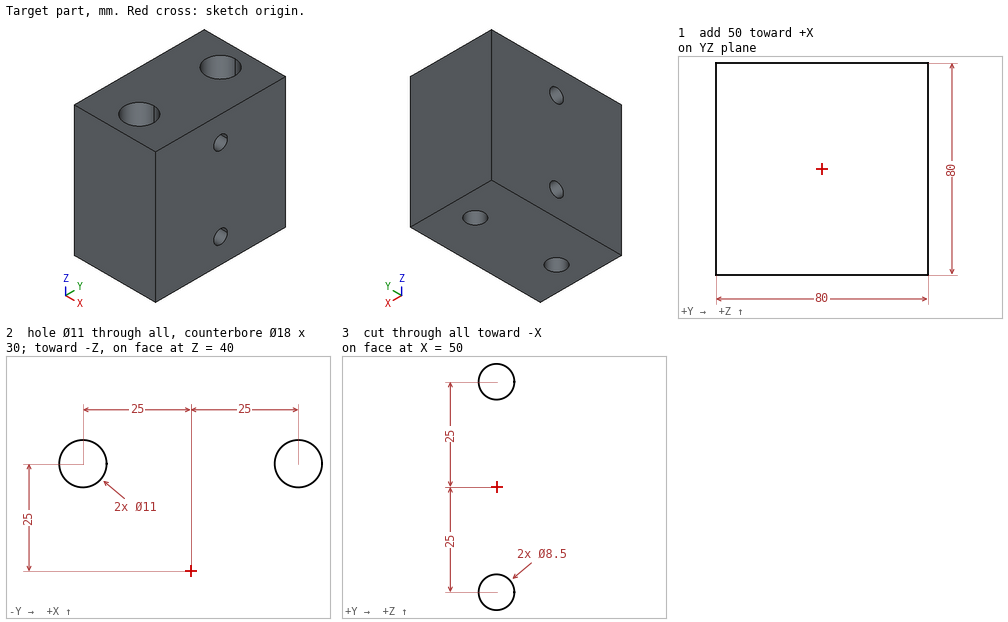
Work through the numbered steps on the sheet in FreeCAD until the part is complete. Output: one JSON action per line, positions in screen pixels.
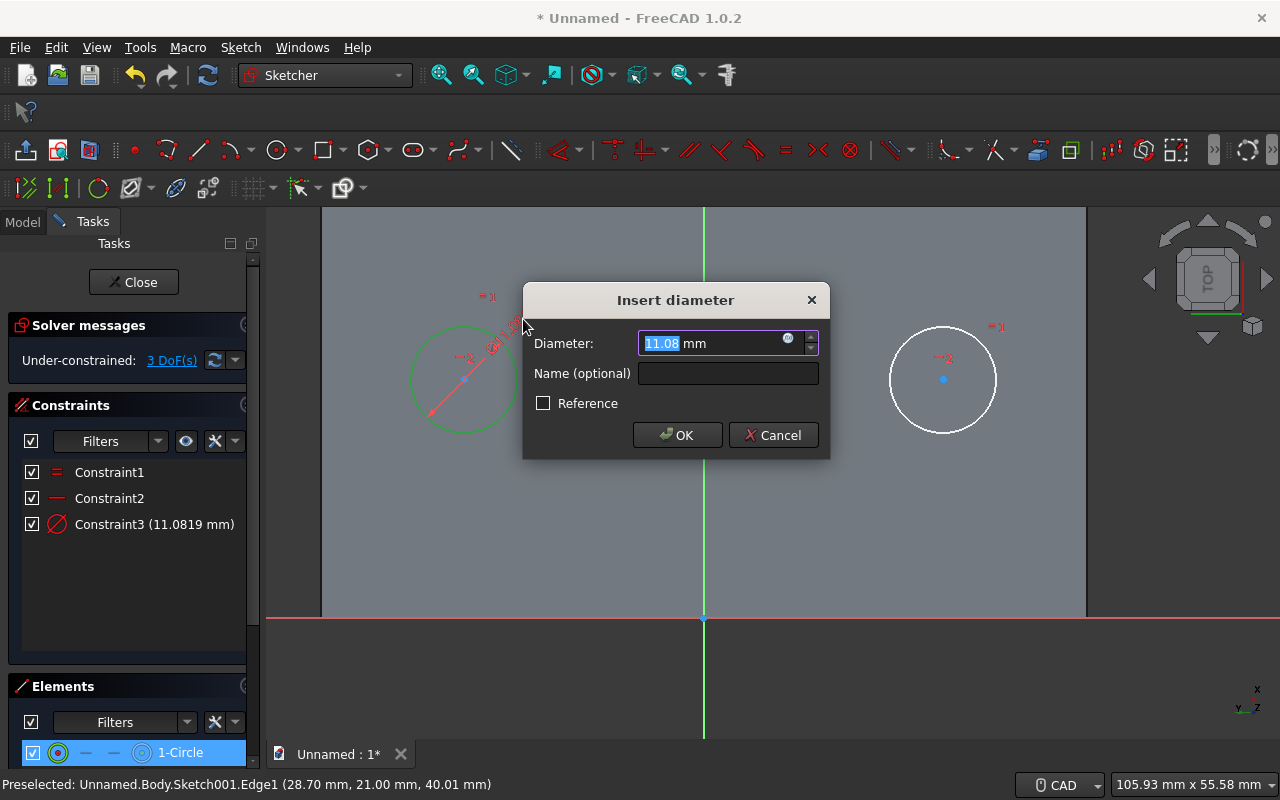
{"action": "type", "text": "11"}
{"action": "key", "text": "Return"}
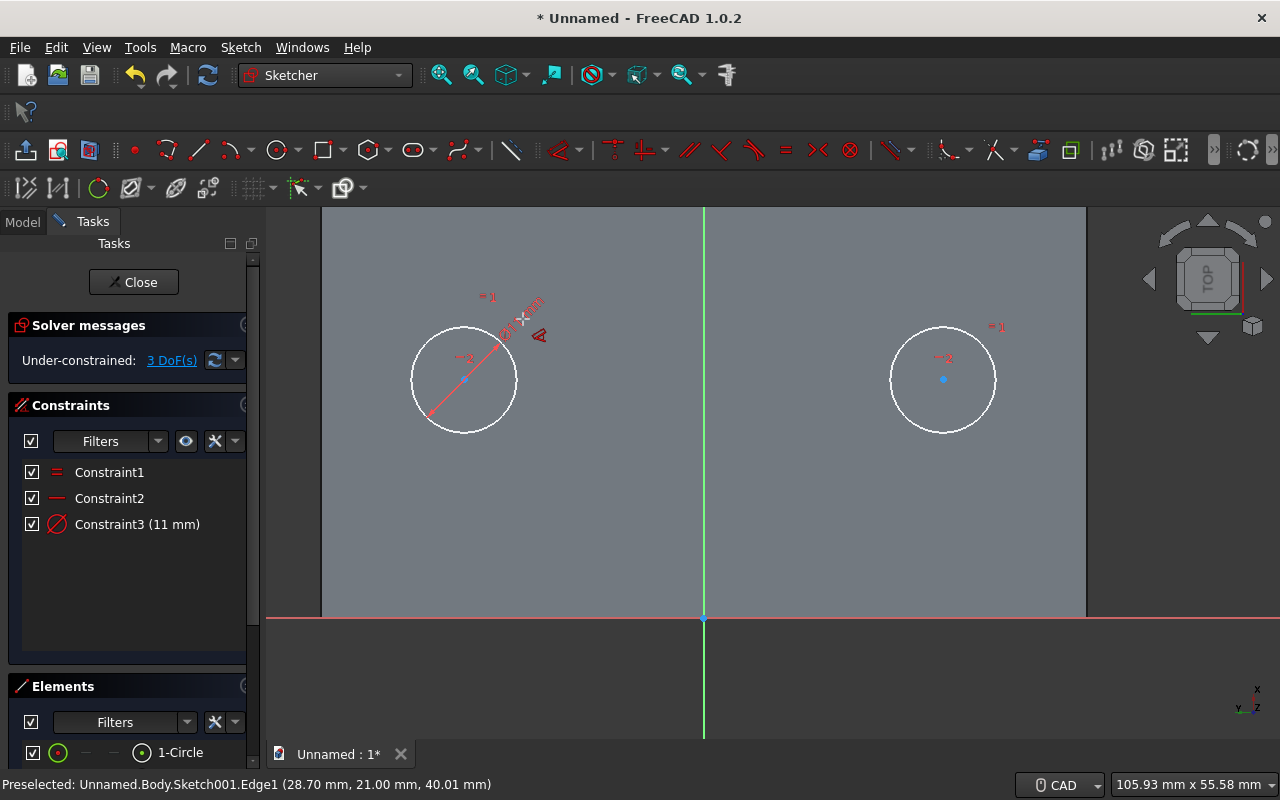
{"action": "left_click", "coordinate": [464, 380]}
{"action": "left_click", "coordinate": [584, 652]}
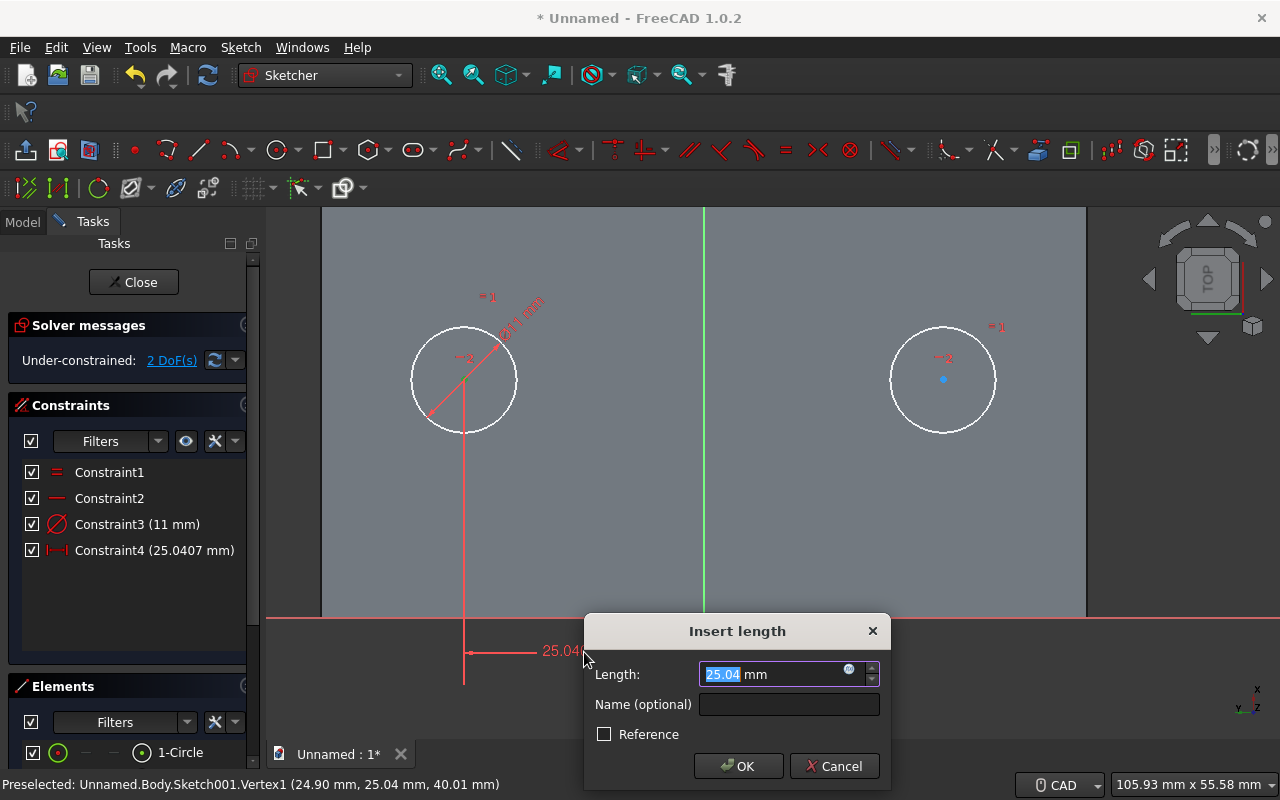
{"action": "type", "text": "25"}
{"action": "key", "text": "Return"}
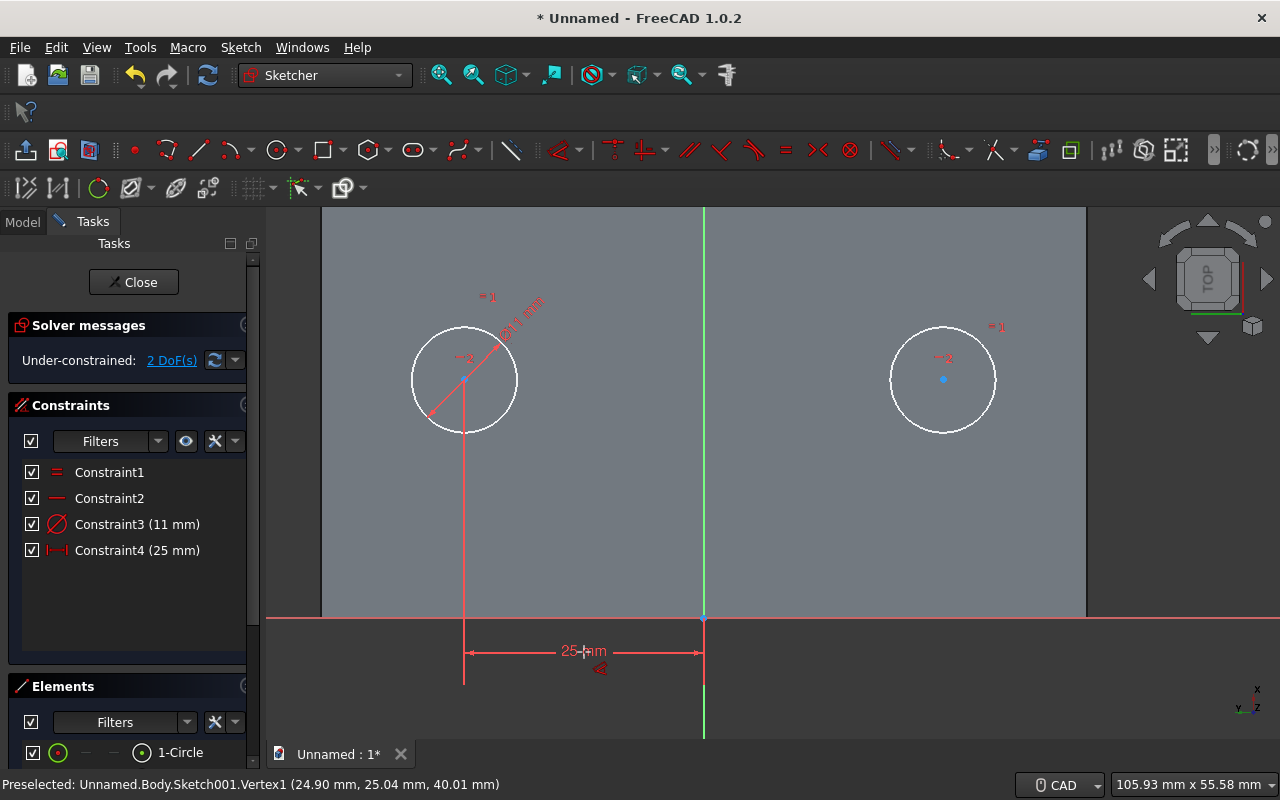
{"action": "left_click", "coordinate": [464, 380]}
{"action": "left_click", "coordinate": [430, 499]}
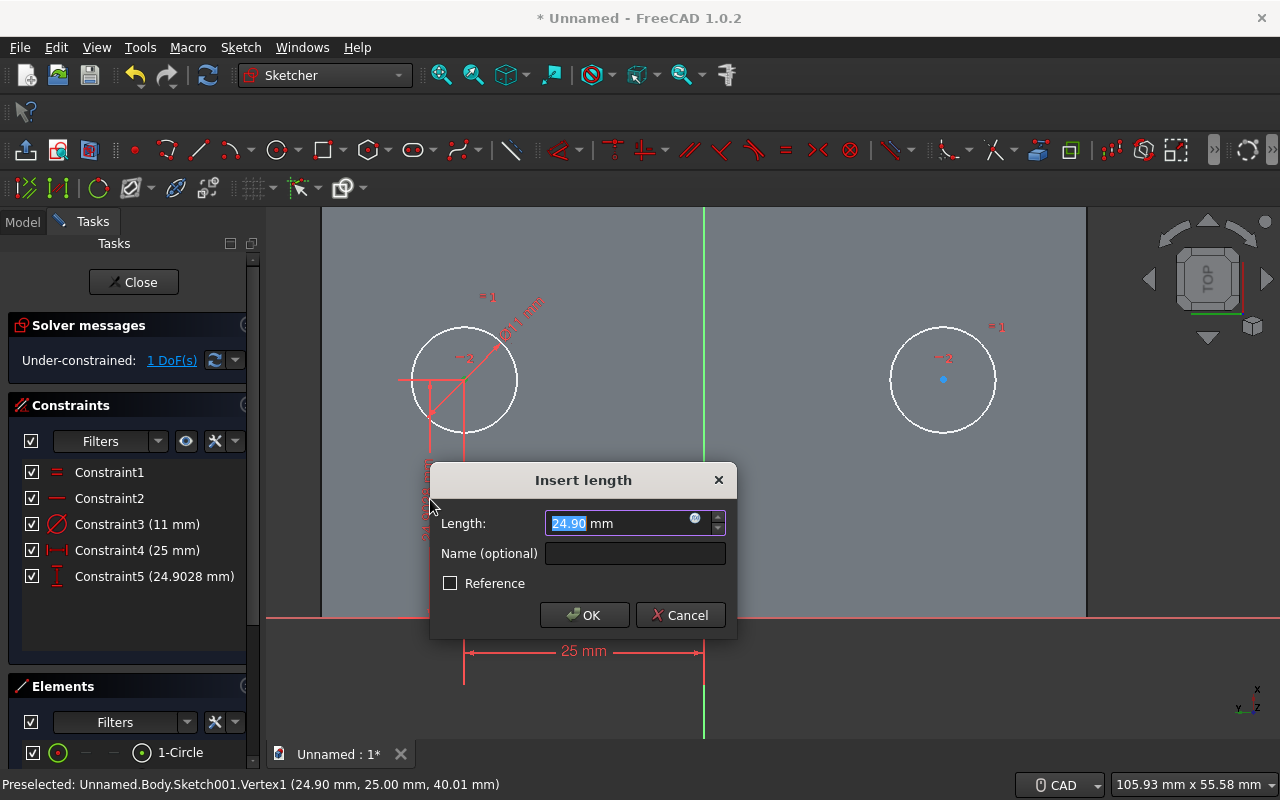
{"action": "type", "text": "25"}
{"action": "key", "text": "Return"}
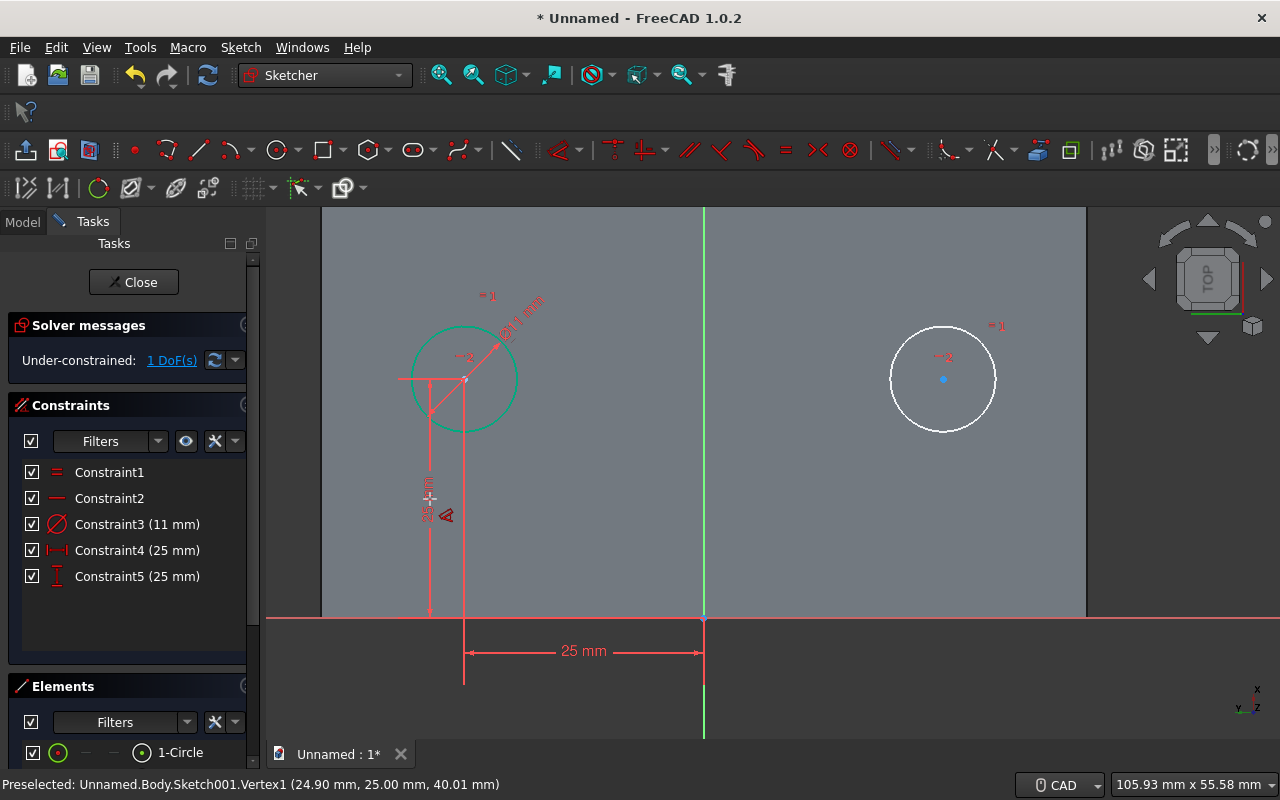
{"action": "left_click", "coordinate": [943, 379]}
{"action": "left_click", "coordinate": [823, 652]}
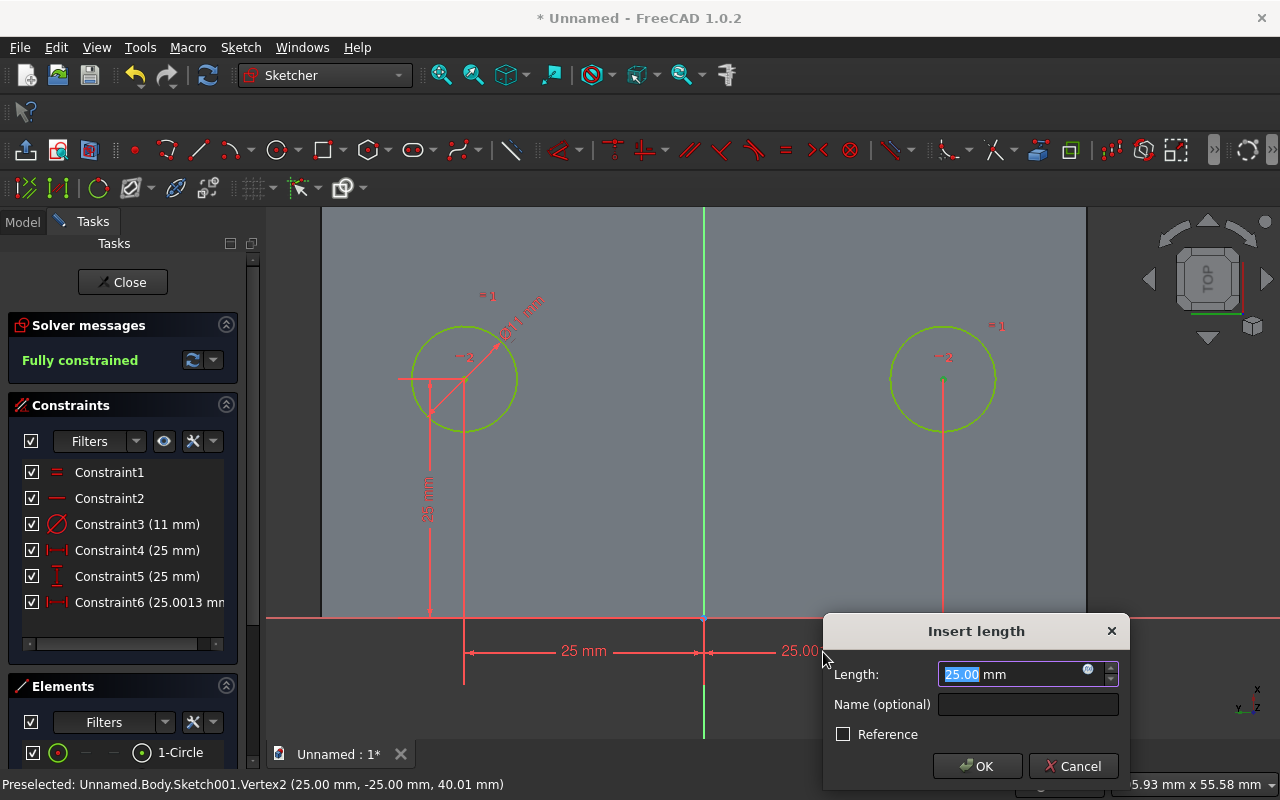
{"action": "type", "text": "25"}
{"action": "key", "text": "Return"}
{"action": "key", "text": "Escape"}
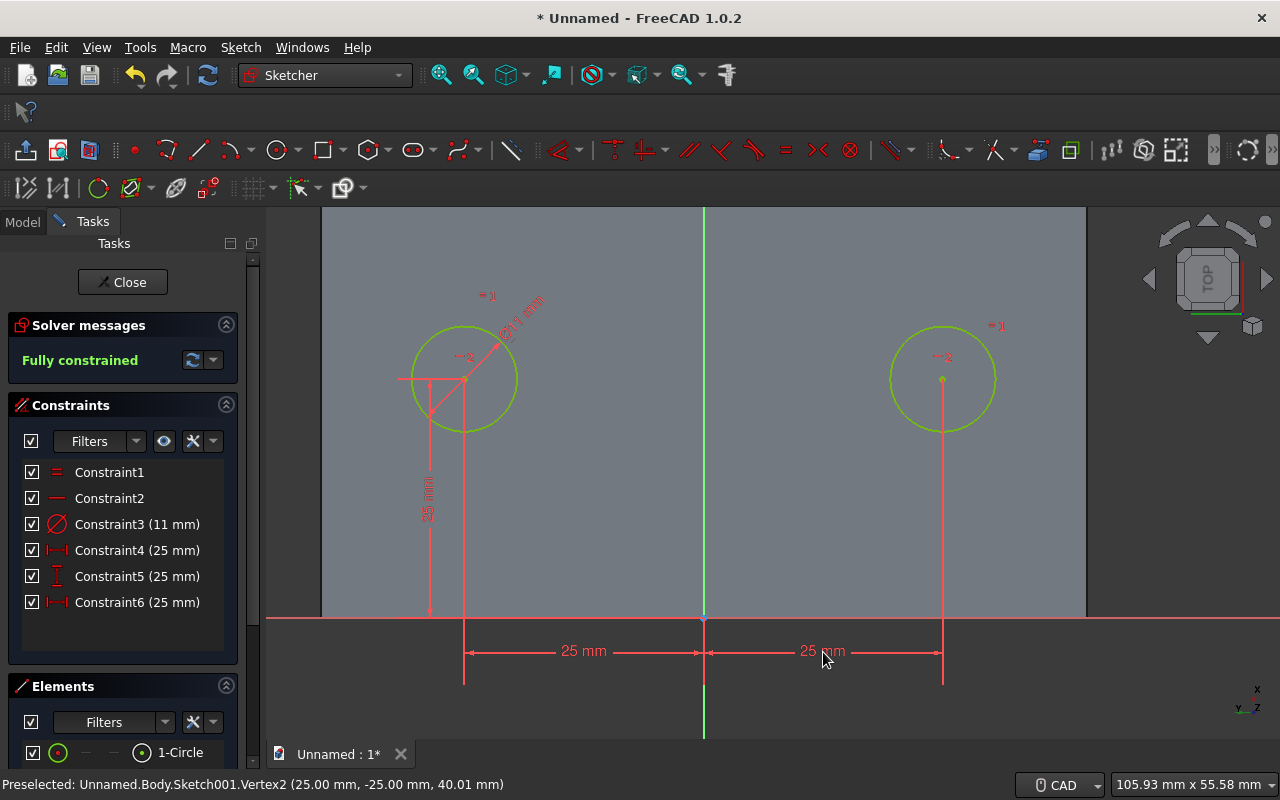
{"action": "left_click", "coordinate": [123, 282]}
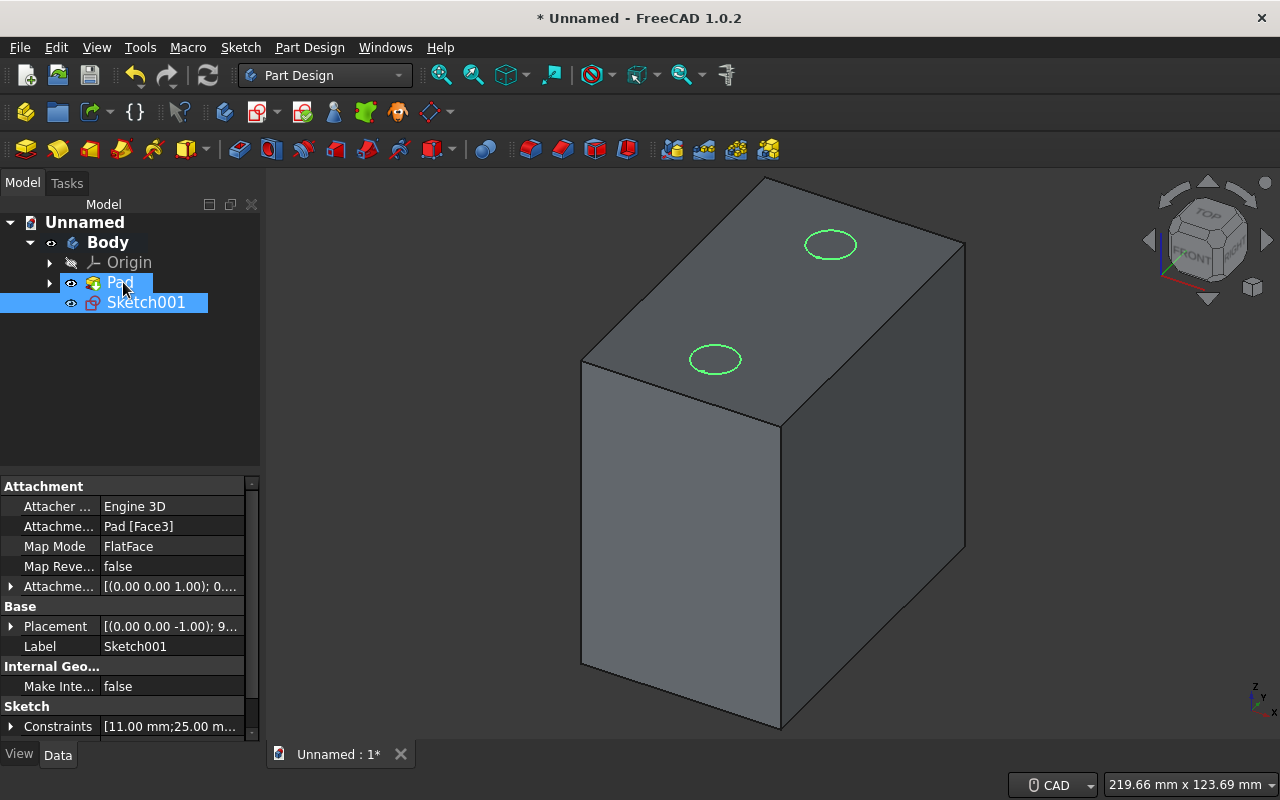
{"action": "left_click", "coordinate": [272, 150]}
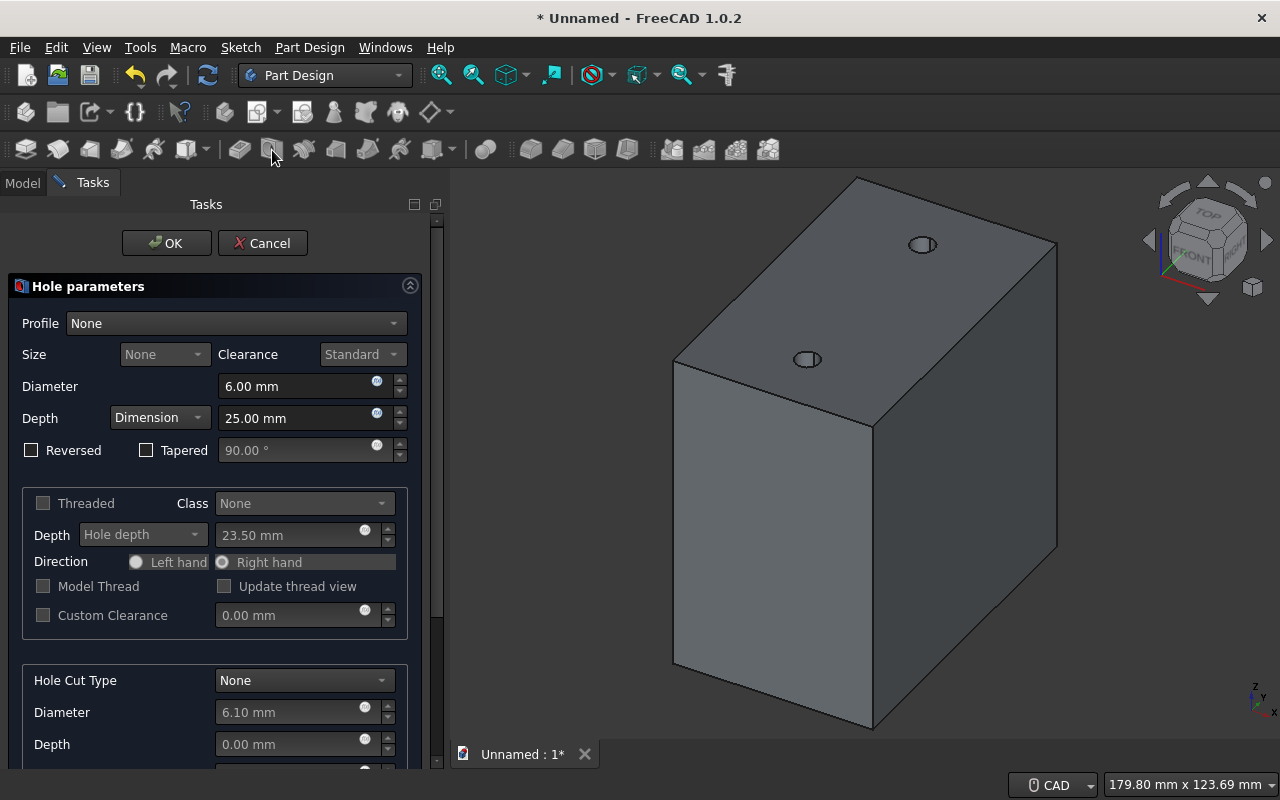
{"action": "triple_click", "coordinate": [305, 386]}